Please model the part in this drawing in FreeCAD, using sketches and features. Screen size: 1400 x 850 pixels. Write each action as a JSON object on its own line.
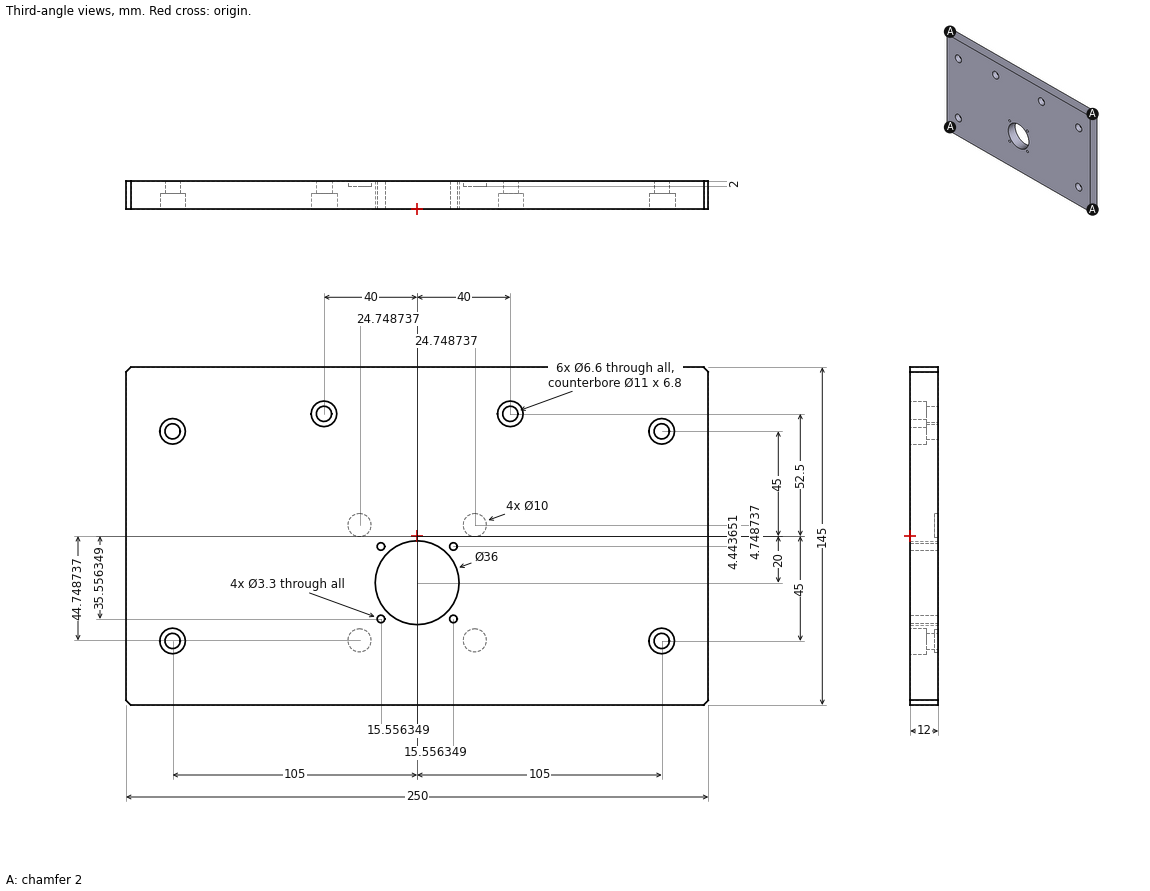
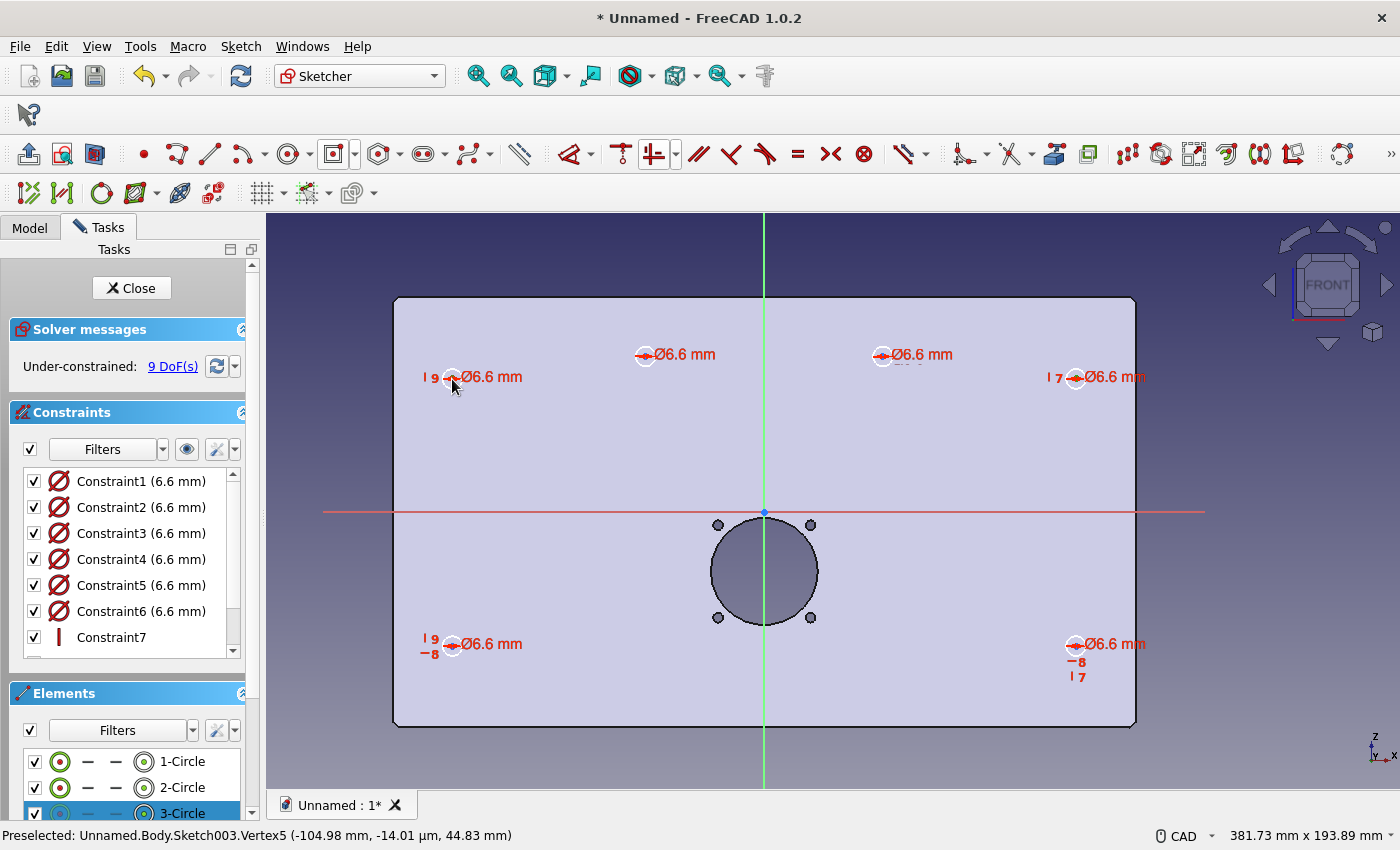
{"action": "left_click", "coordinate": [676, 154]}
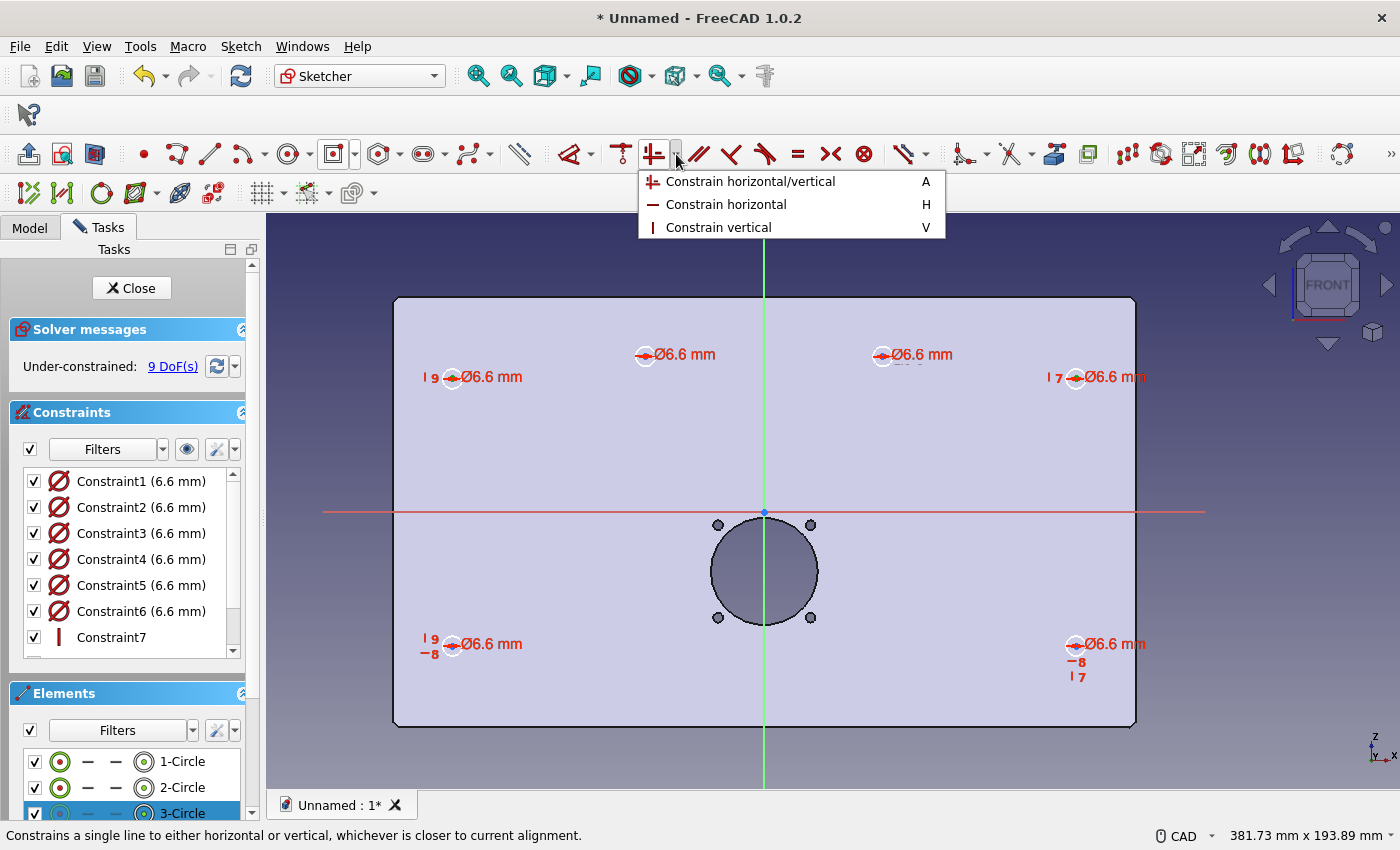
{"action": "left_click", "coordinate": [792, 204]}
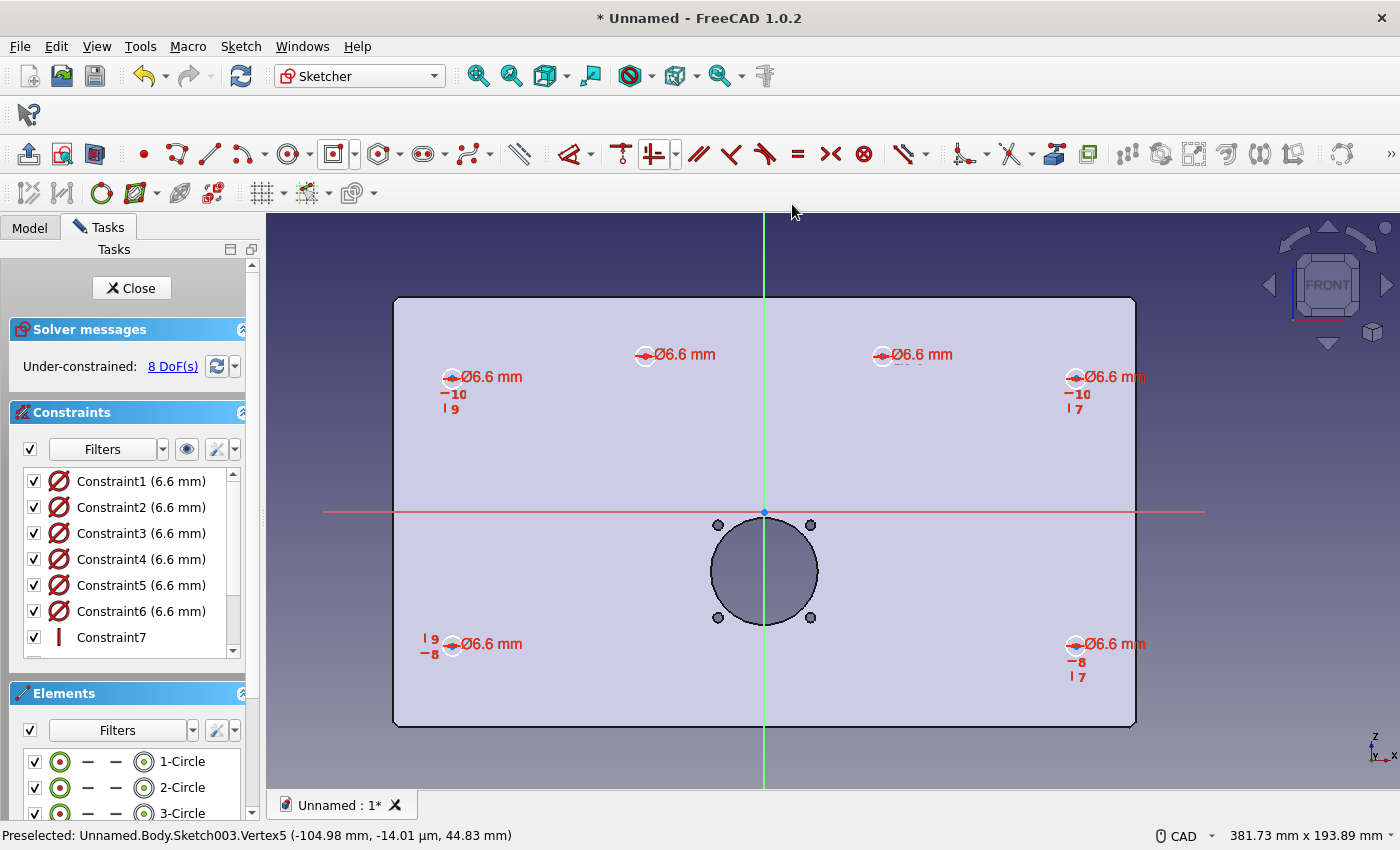
{"action": "left_click", "coordinate": [883, 357]}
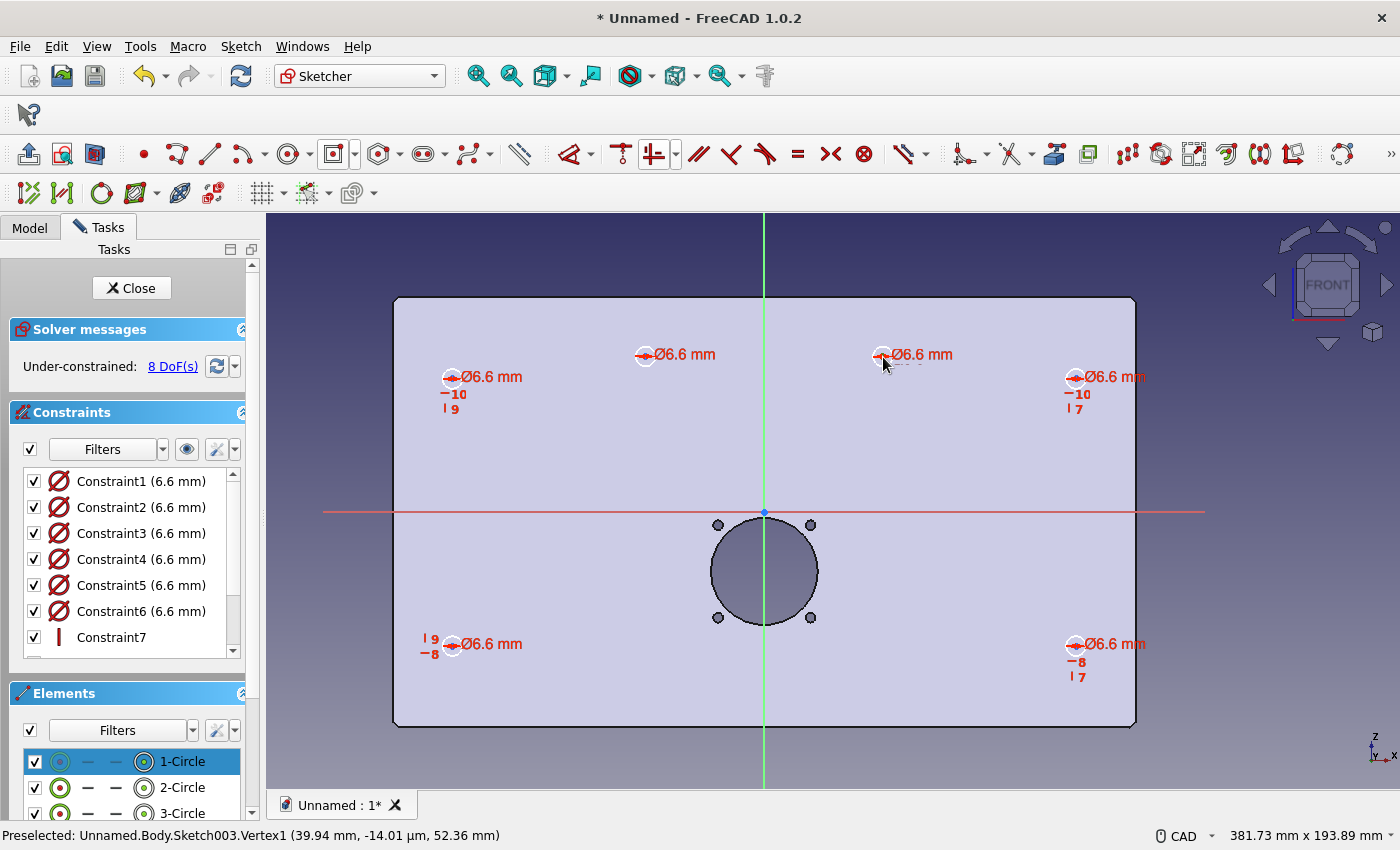
{"action": "left_click", "coordinate": [646, 356]}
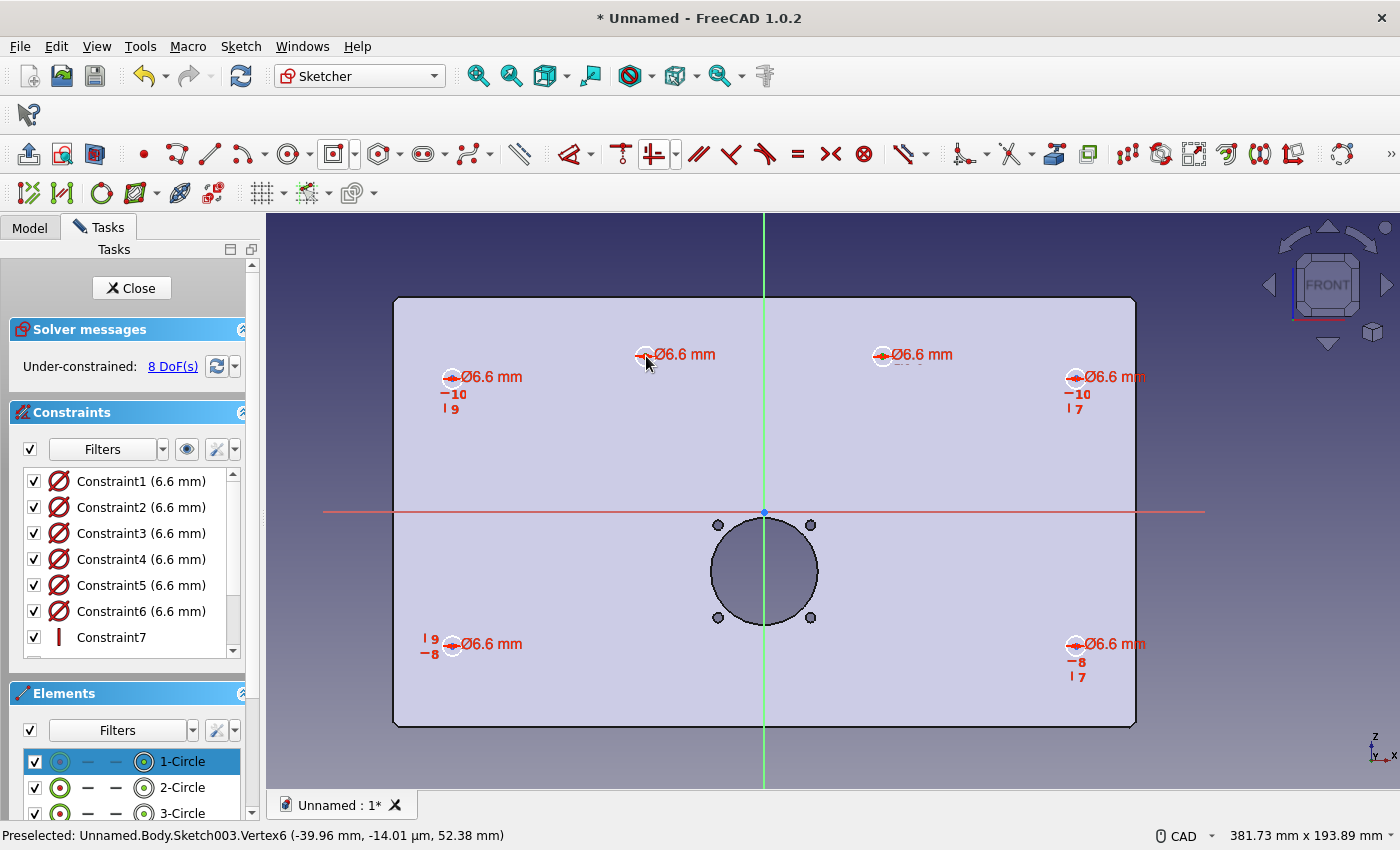
{"action": "key", "text": "h"}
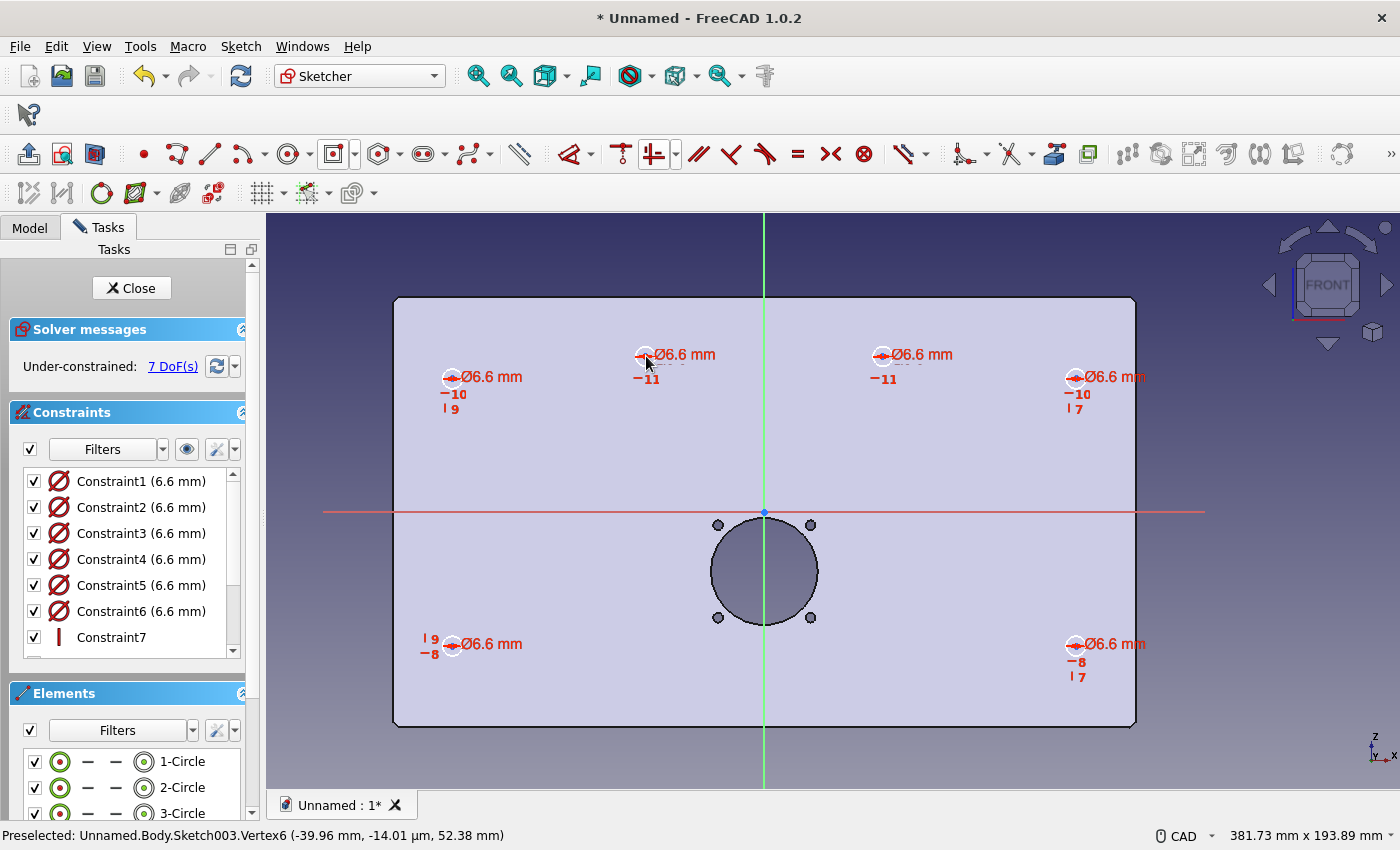
{"action": "left_click", "coordinate": [568, 154]}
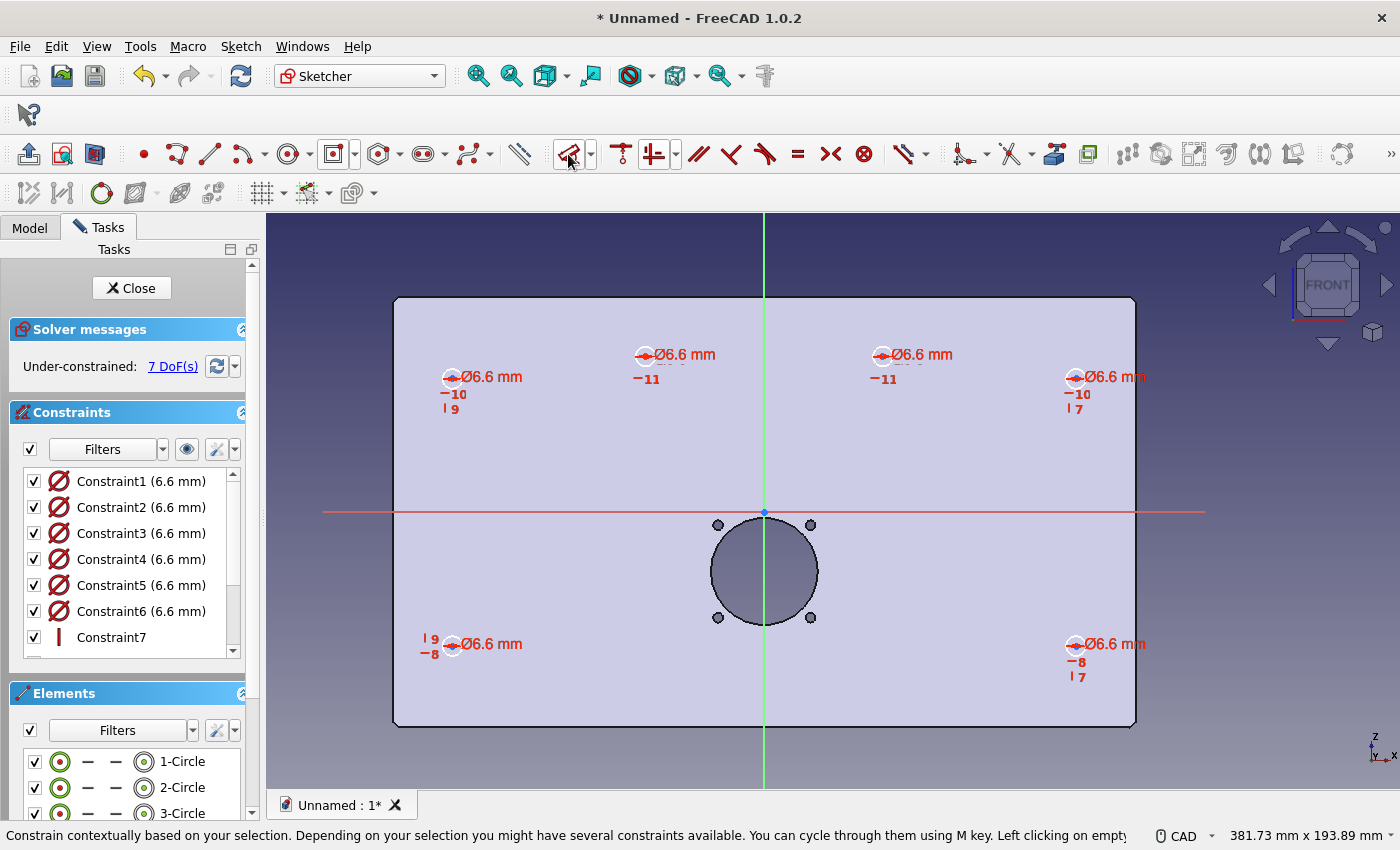
{"action": "left_click", "coordinate": [883, 357]}
{"action": "left_click", "coordinate": [824, 323]}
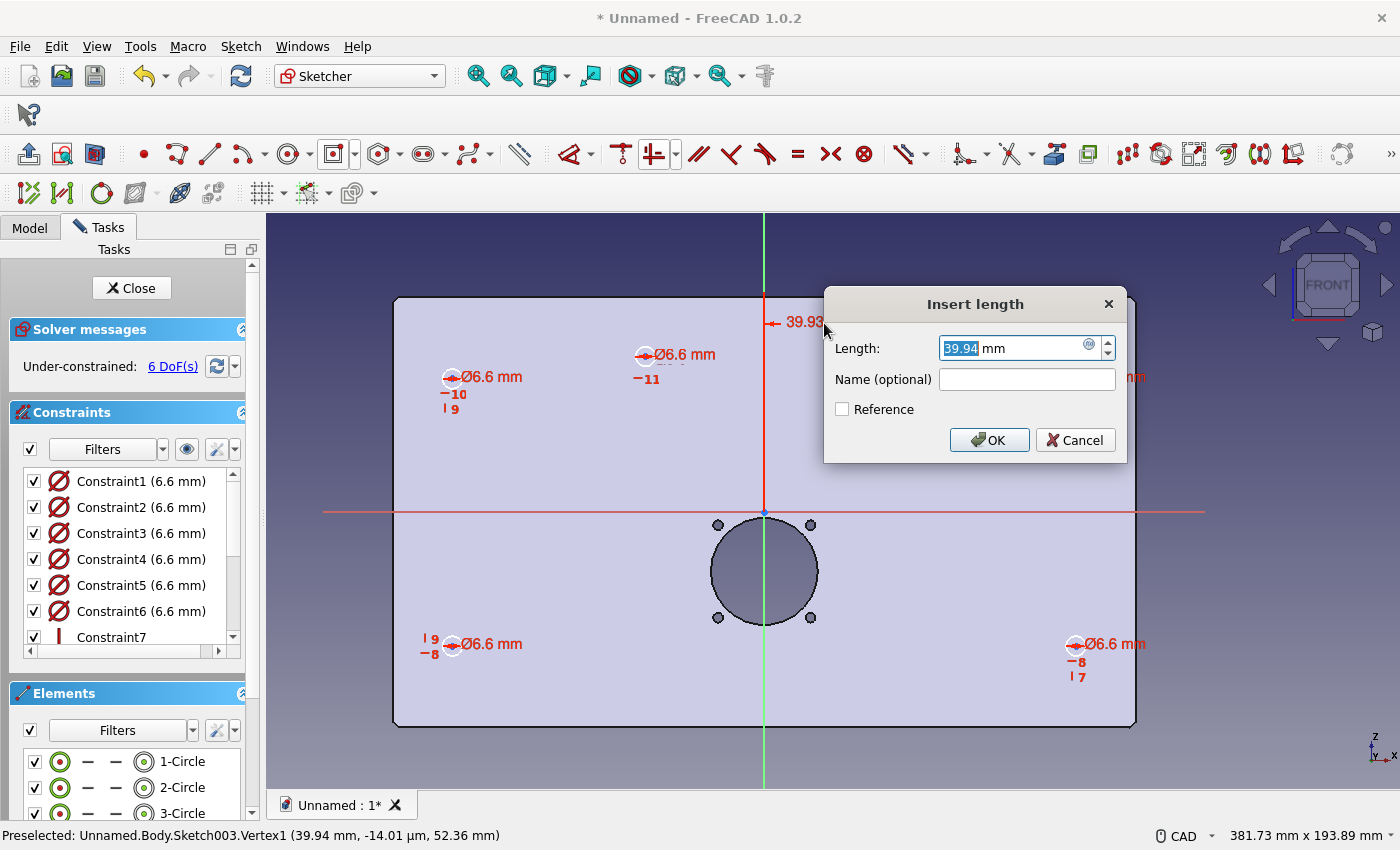
{"action": "type", "text": "40"}
{"action": "key", "text": "Return"}